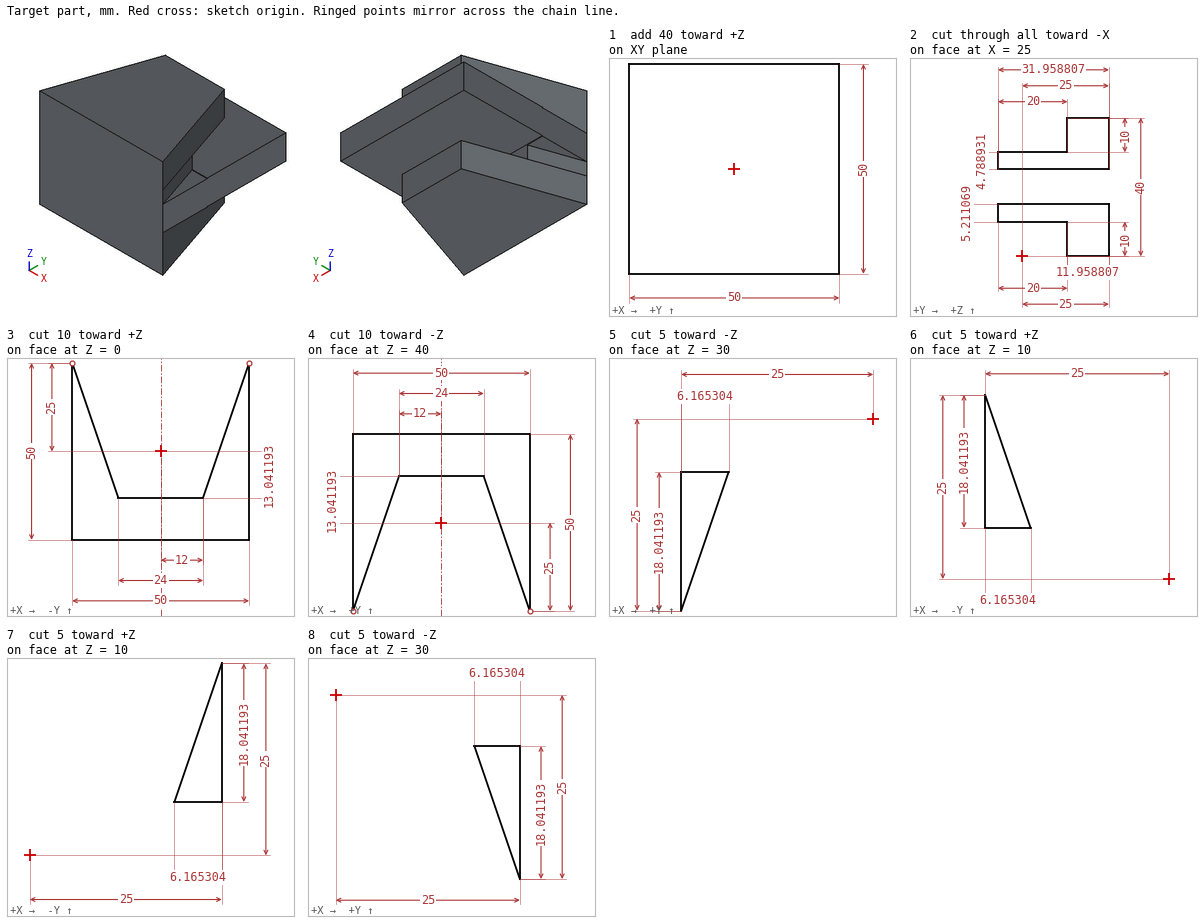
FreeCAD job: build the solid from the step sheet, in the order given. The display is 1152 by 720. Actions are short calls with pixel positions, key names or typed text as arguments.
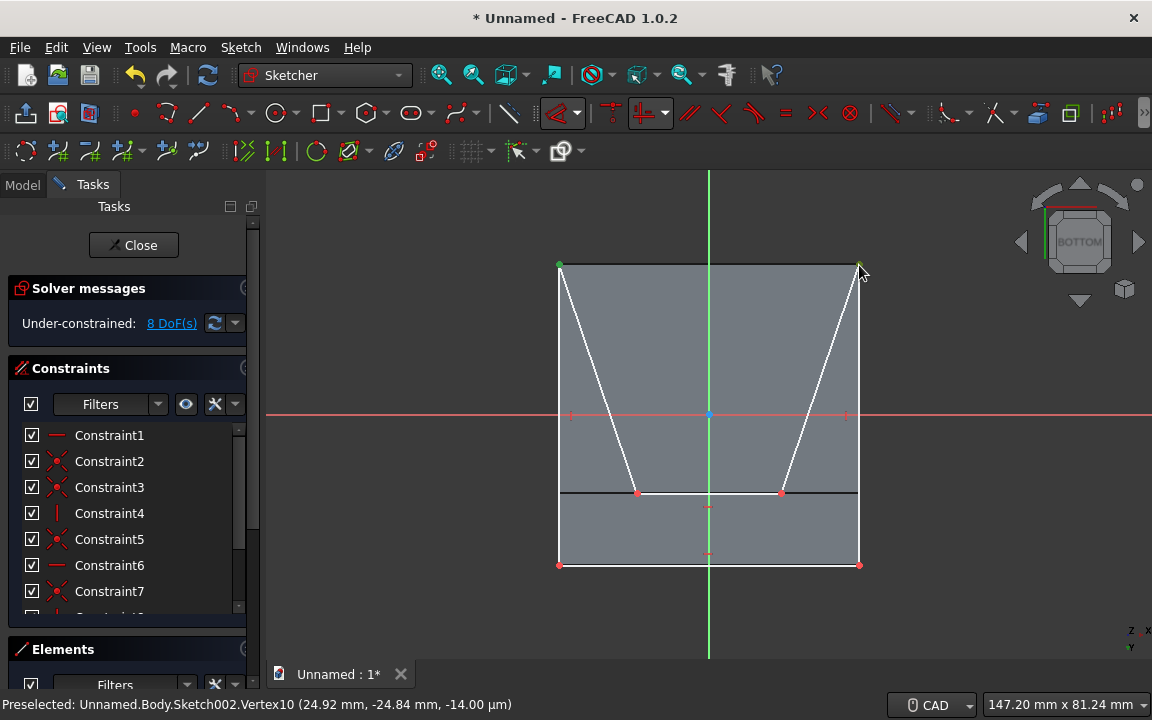
click(709, 600)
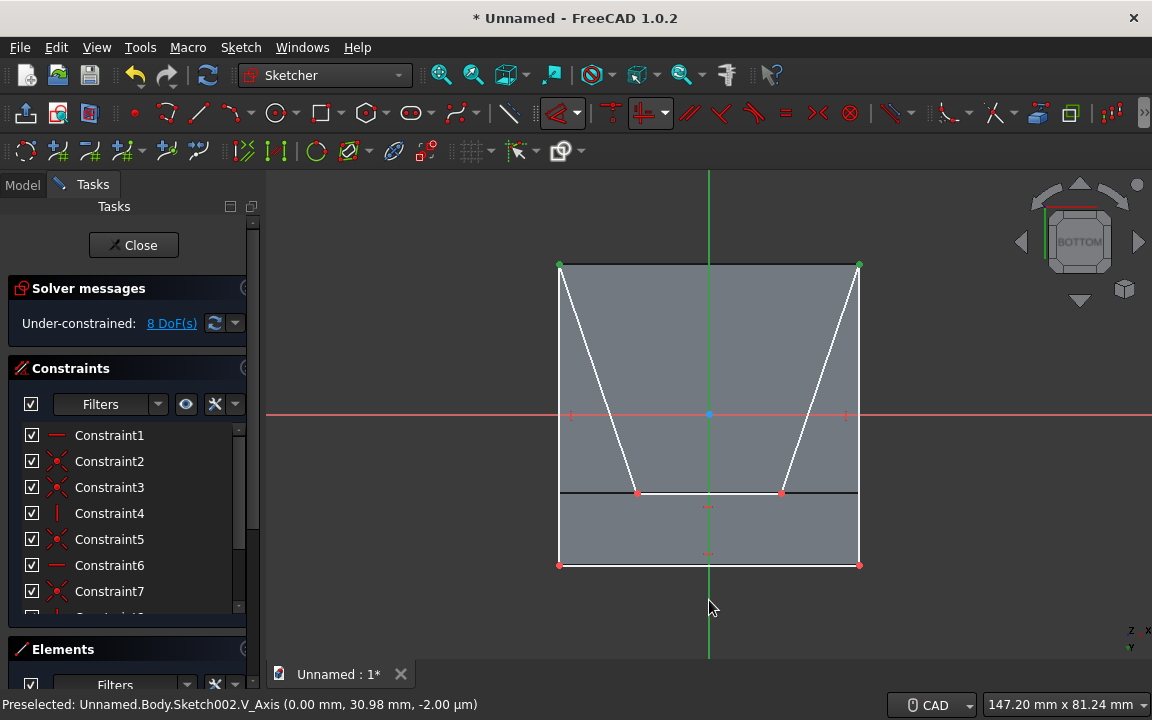
click(818, 114)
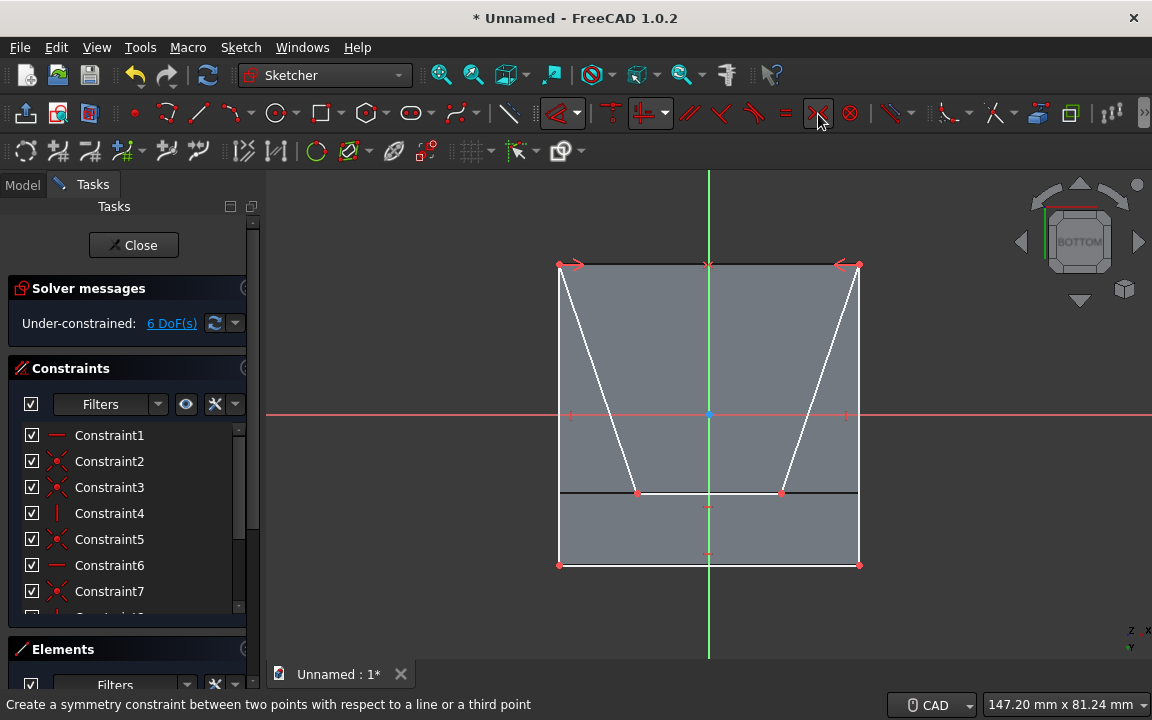
click(738, 494)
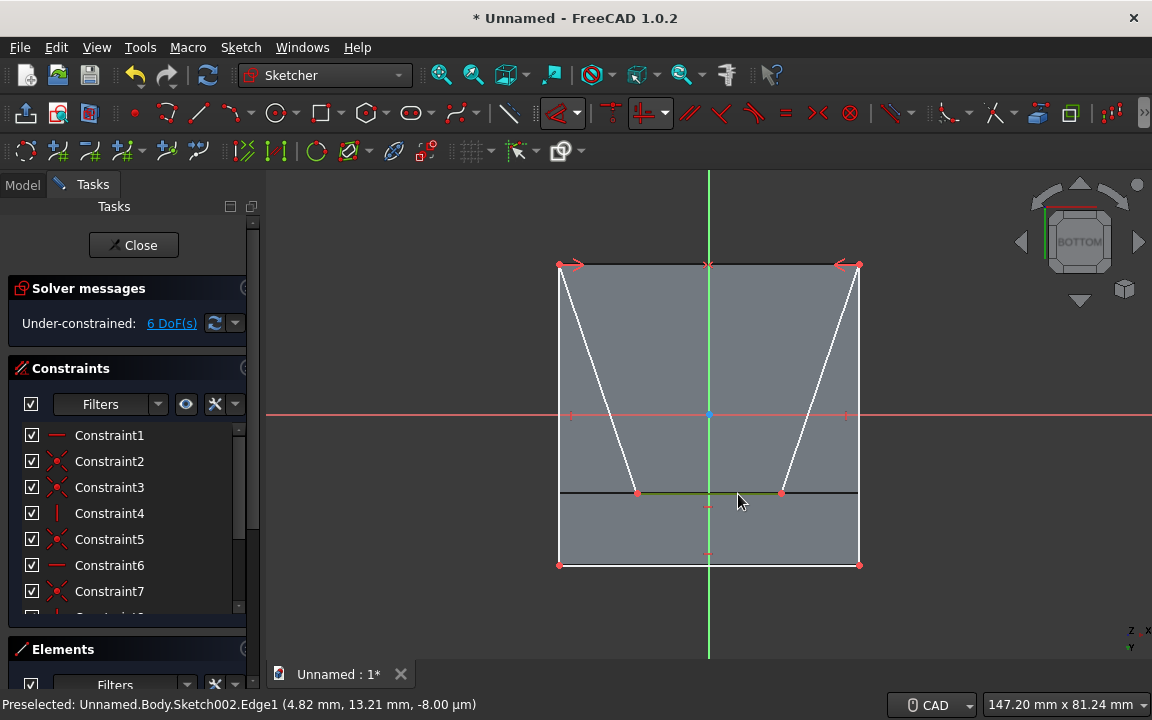
key(l)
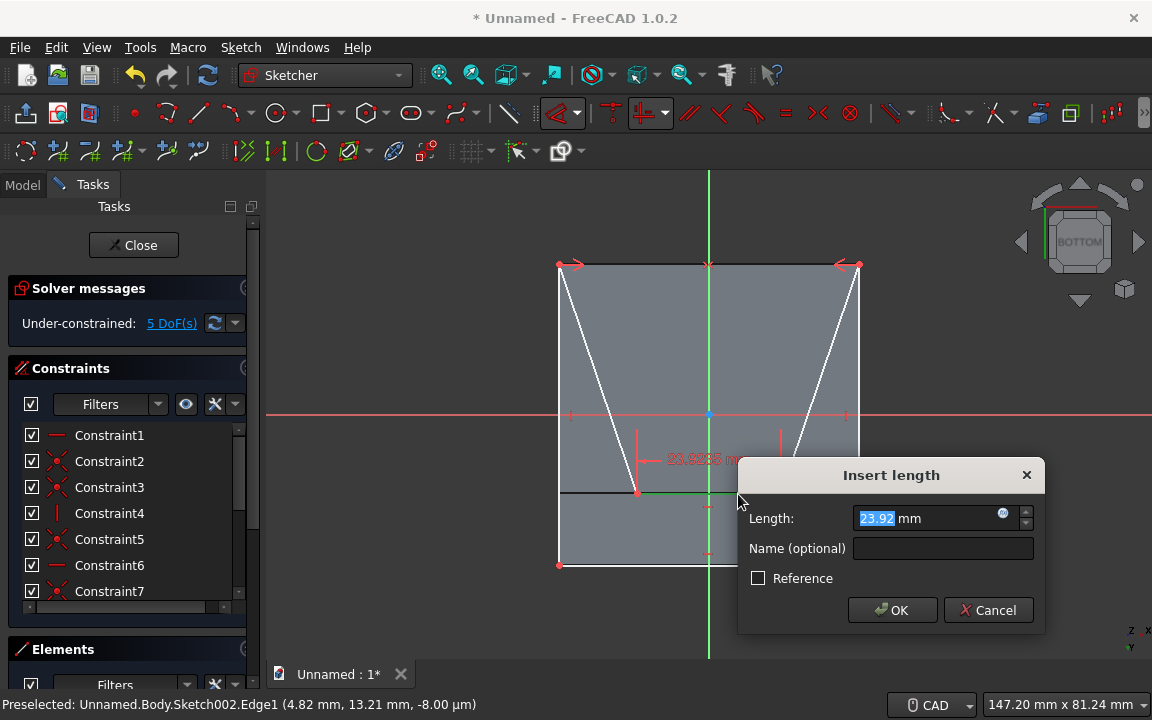
text(24)
key(Return)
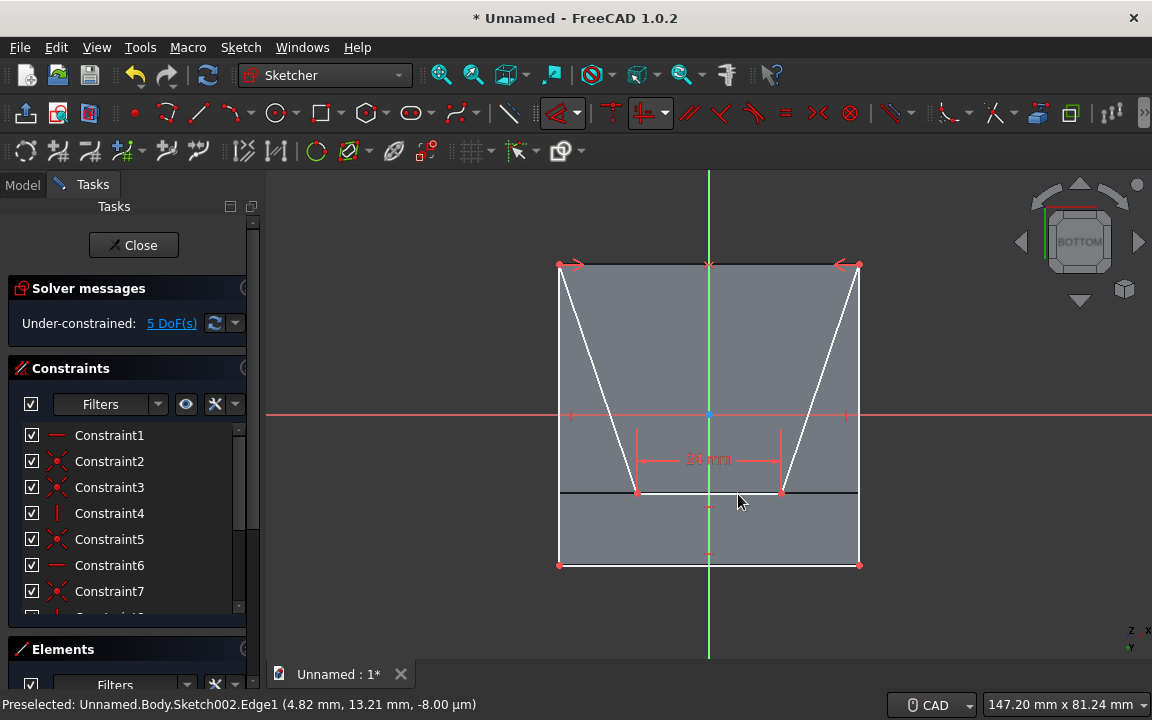
click(559, 355)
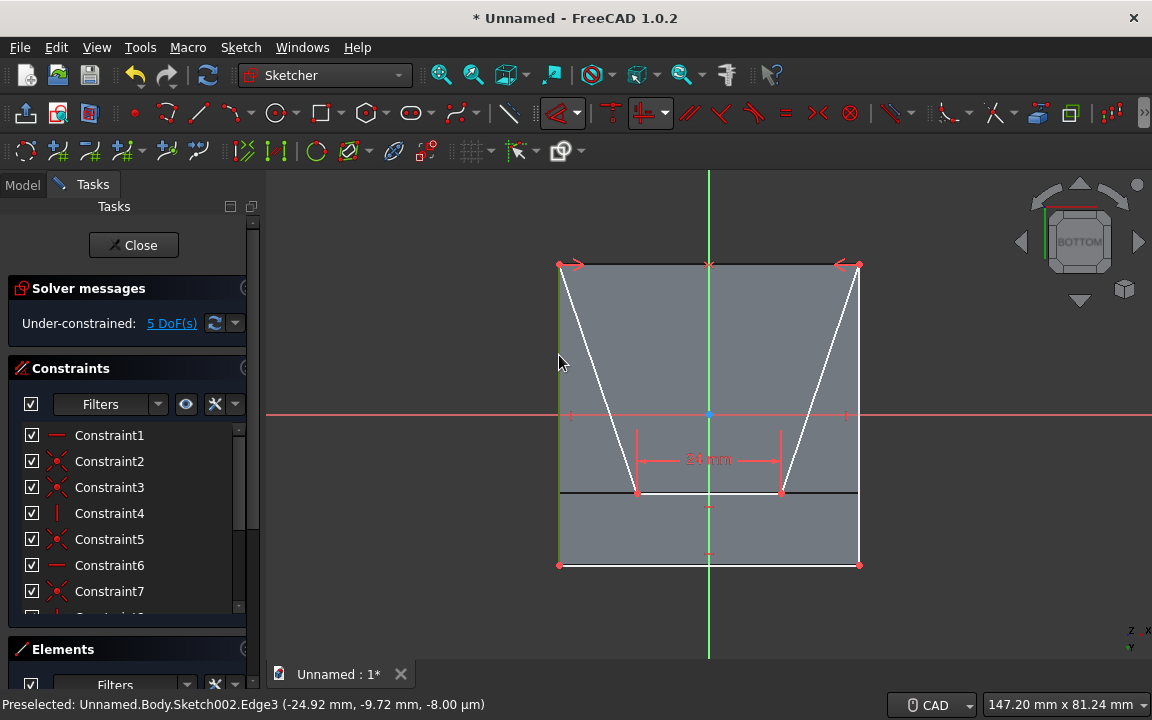
key(i)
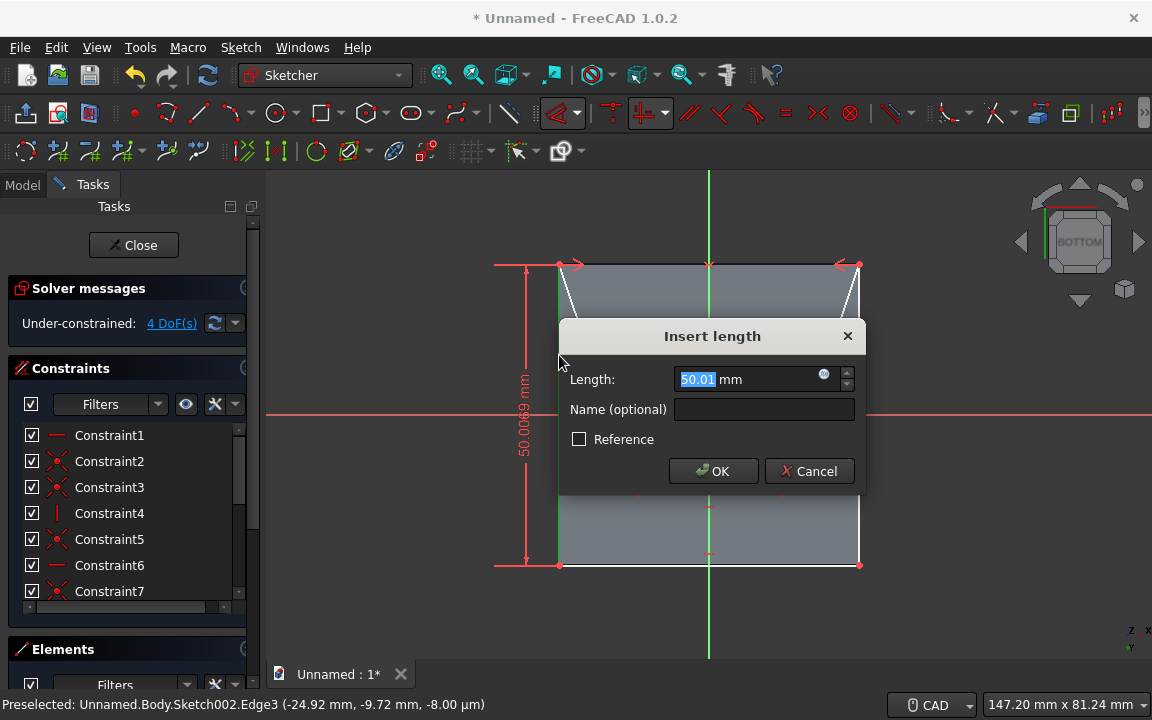
text(50)
key(Return)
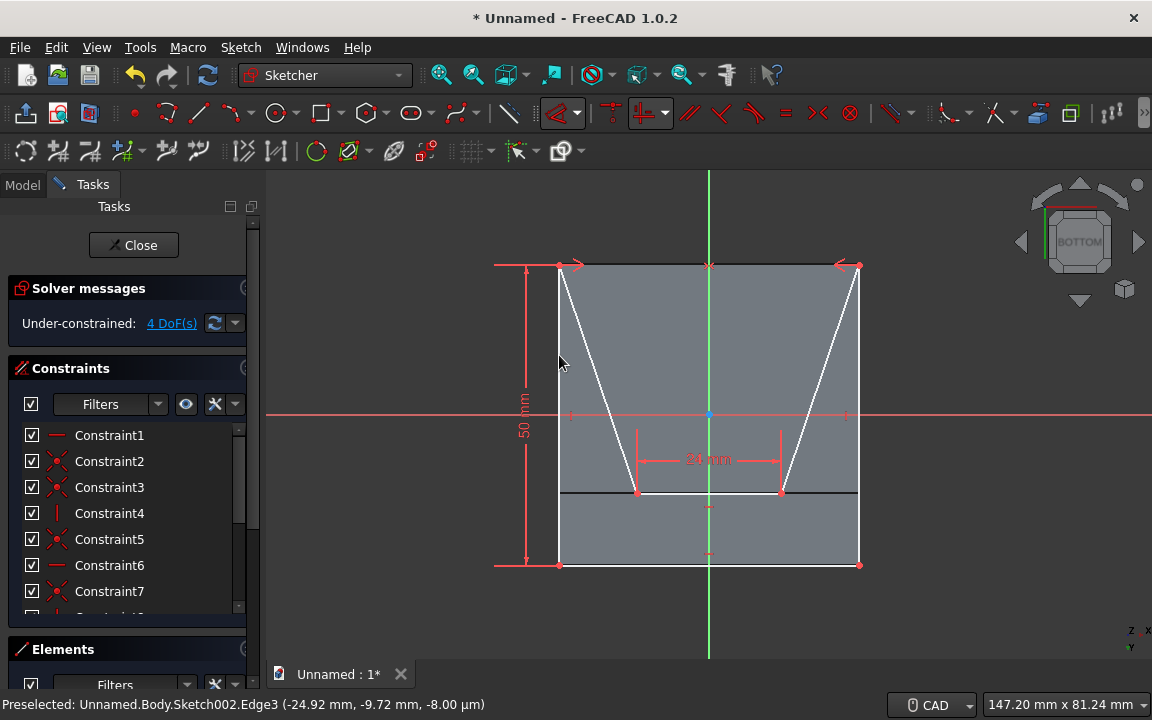
click(649, 566)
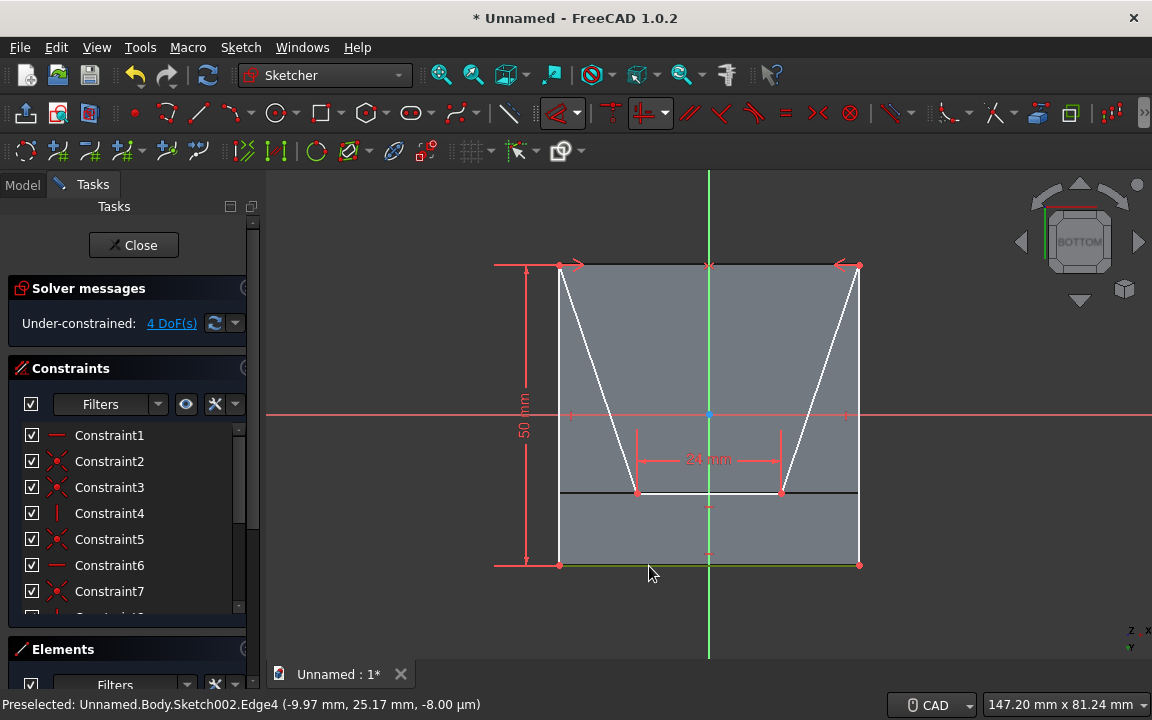
key(l)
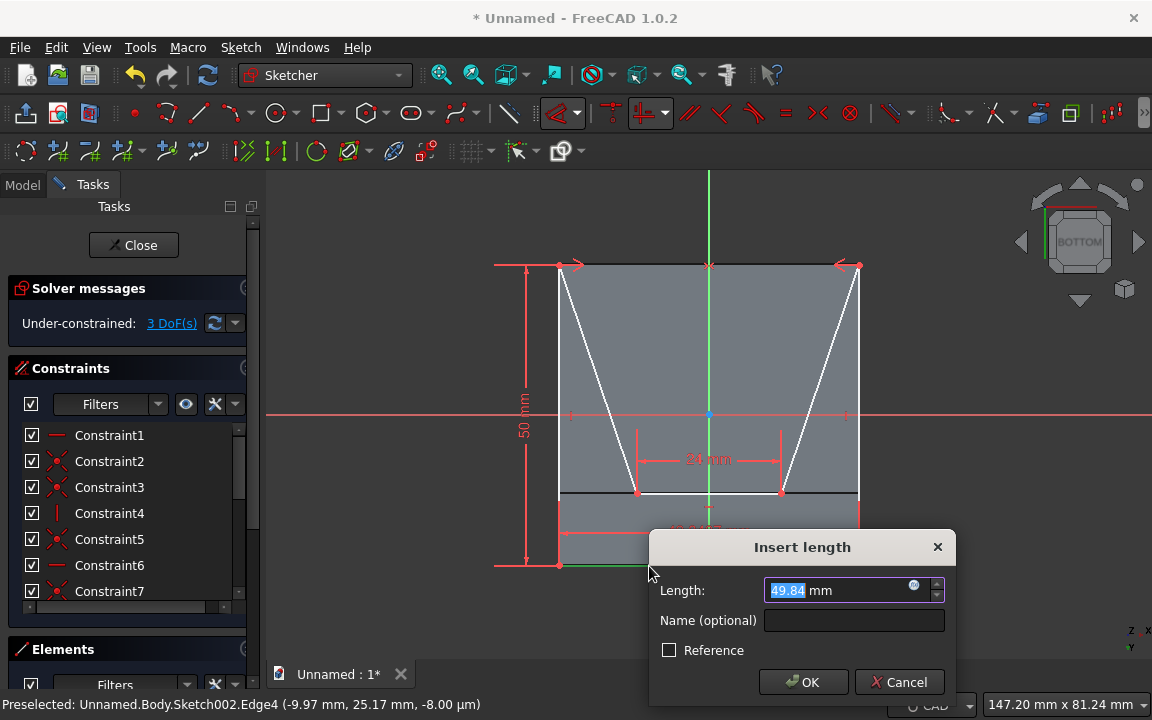
text(50)
key(Return)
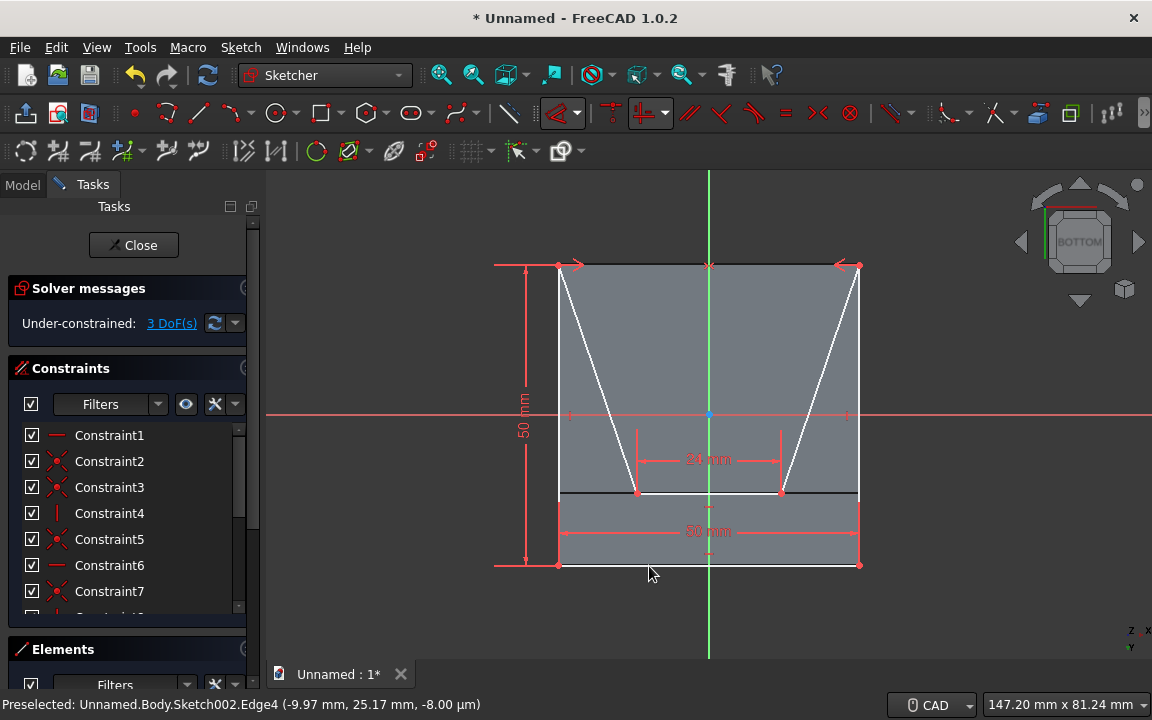
click(781, 494)